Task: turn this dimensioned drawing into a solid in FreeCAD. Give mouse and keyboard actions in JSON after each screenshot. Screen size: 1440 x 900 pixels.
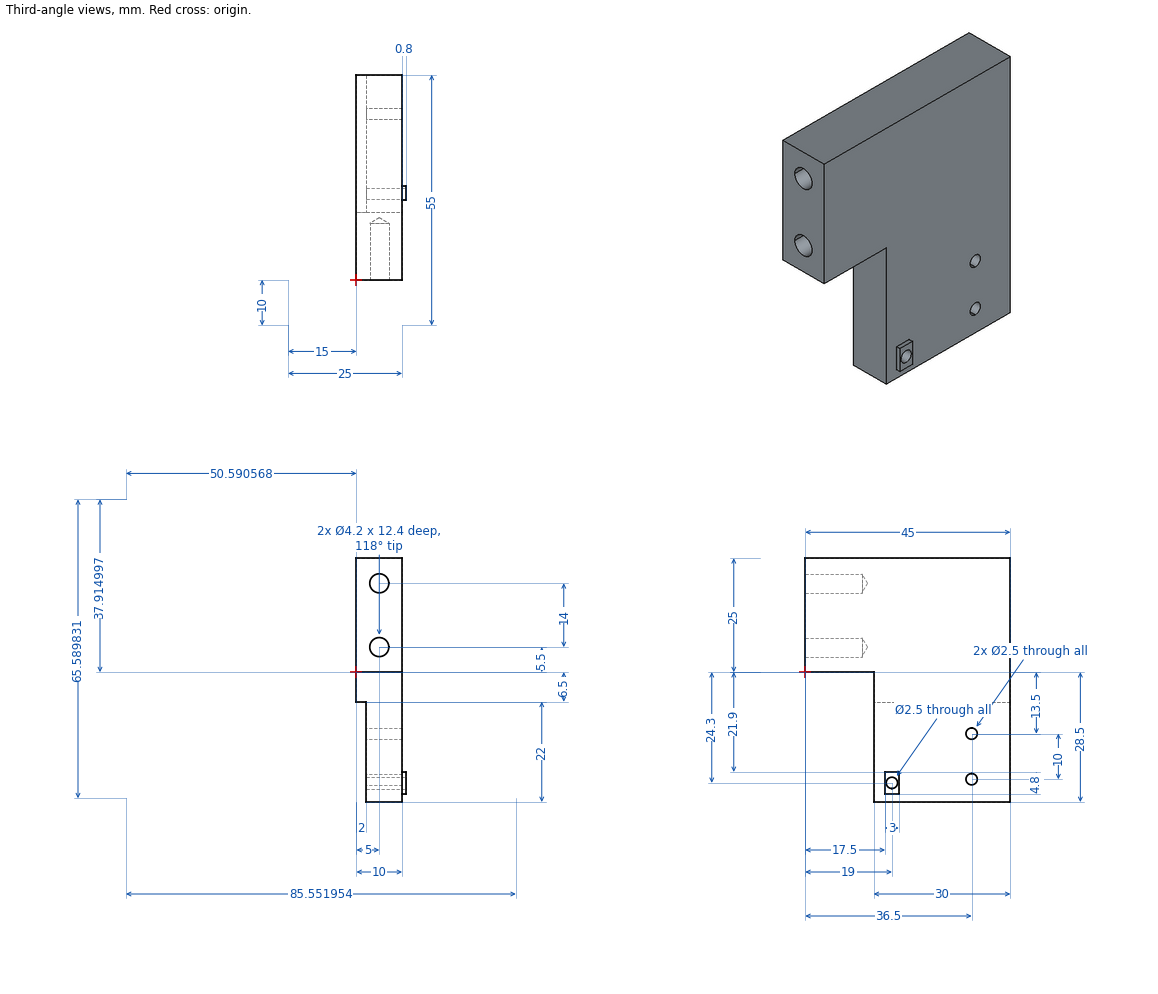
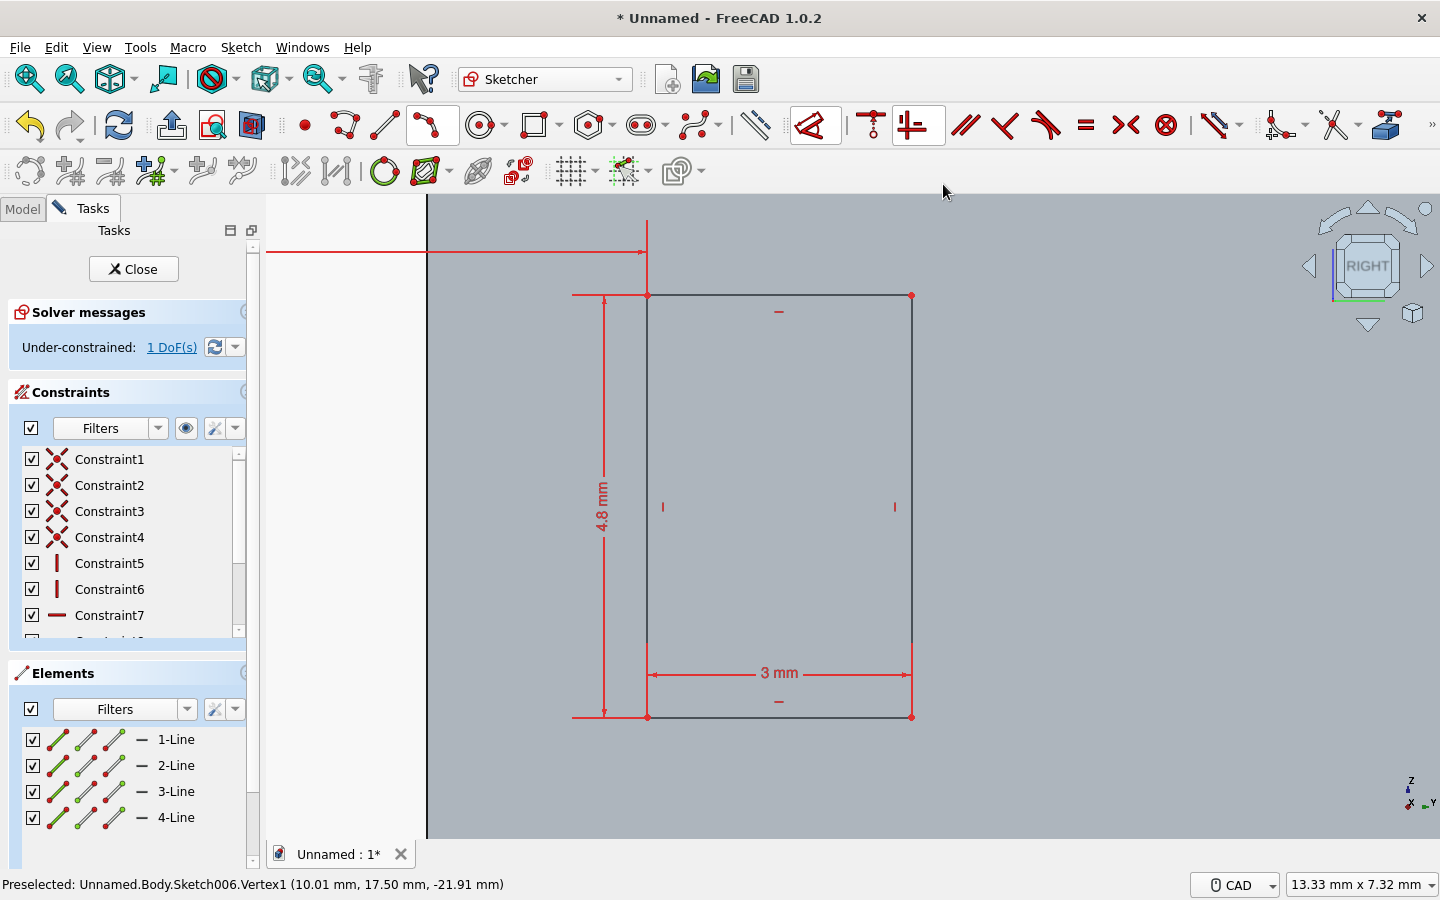
{"action": "left_click", "coordinate": [647, 295]}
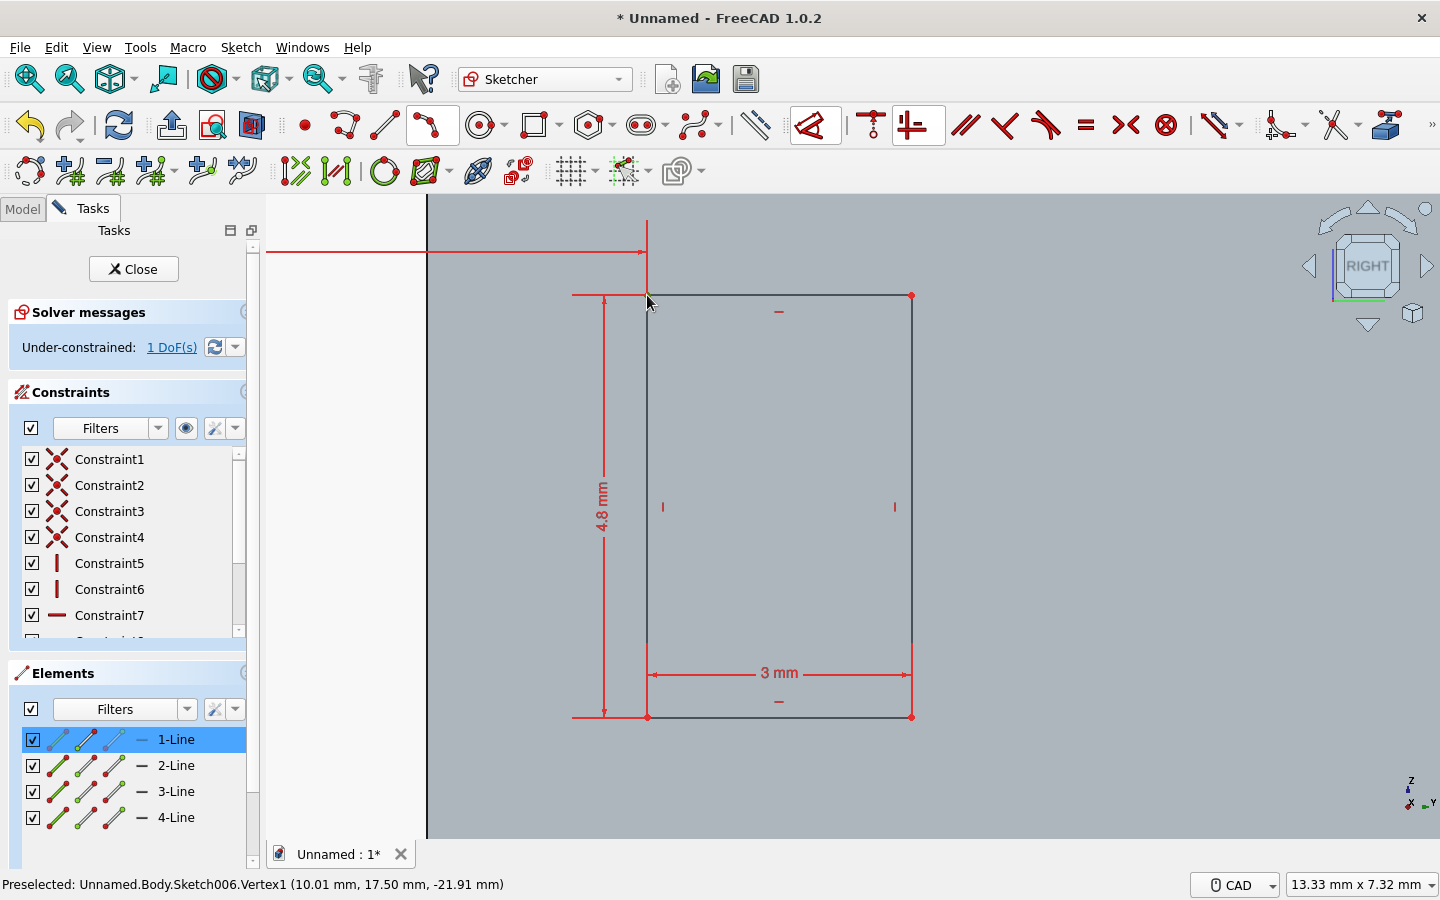
{"action": "key", "text": "i"}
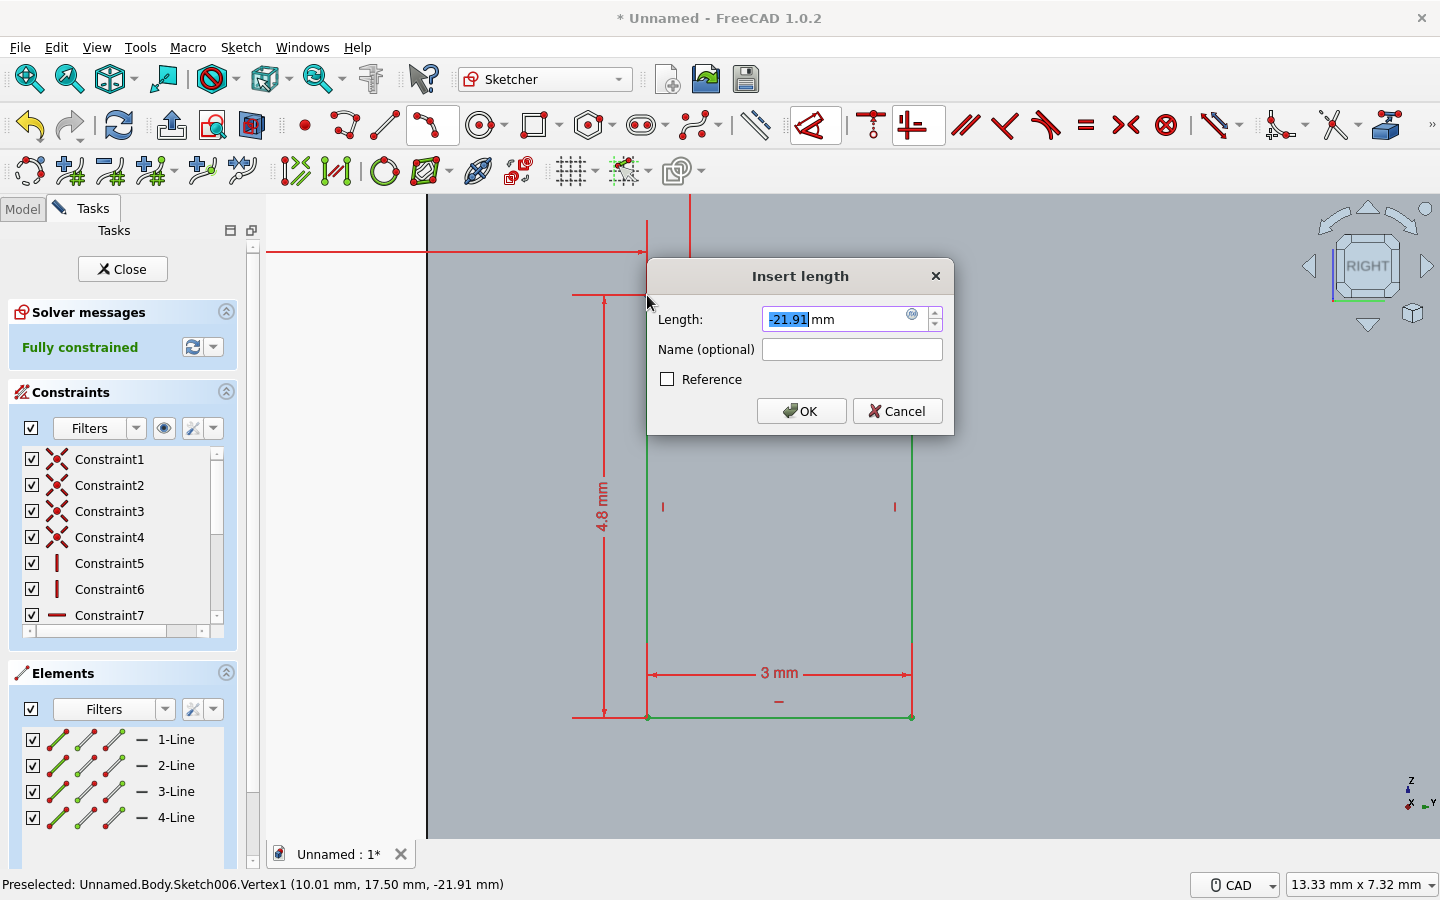
{"action": "type", "text": "-21.9"}
{"action": "key", "text": "Return"}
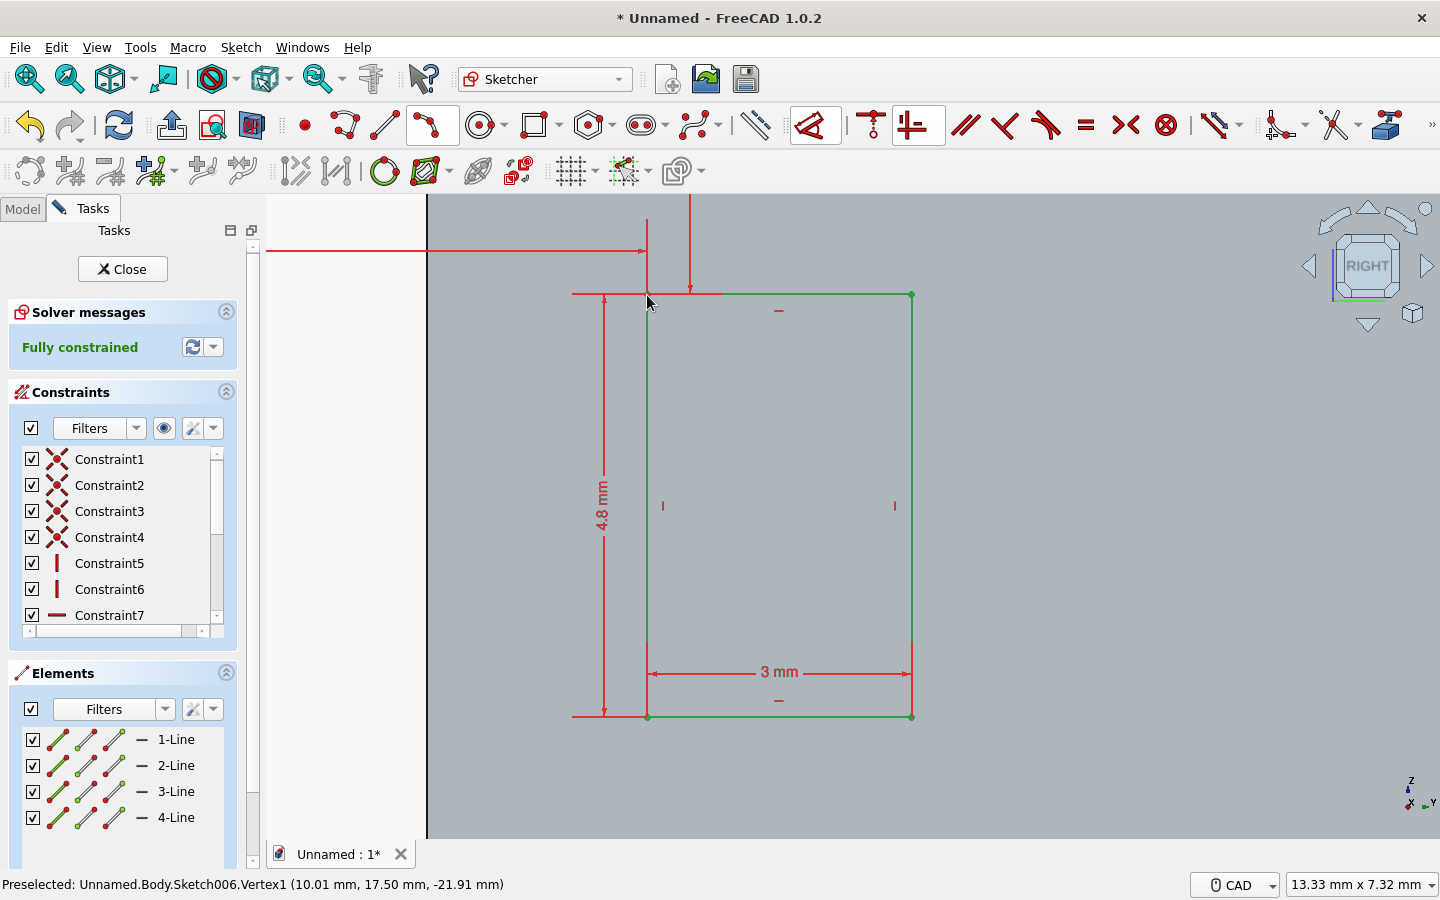
{"action": "left_click", "coordinate": [123, 269]}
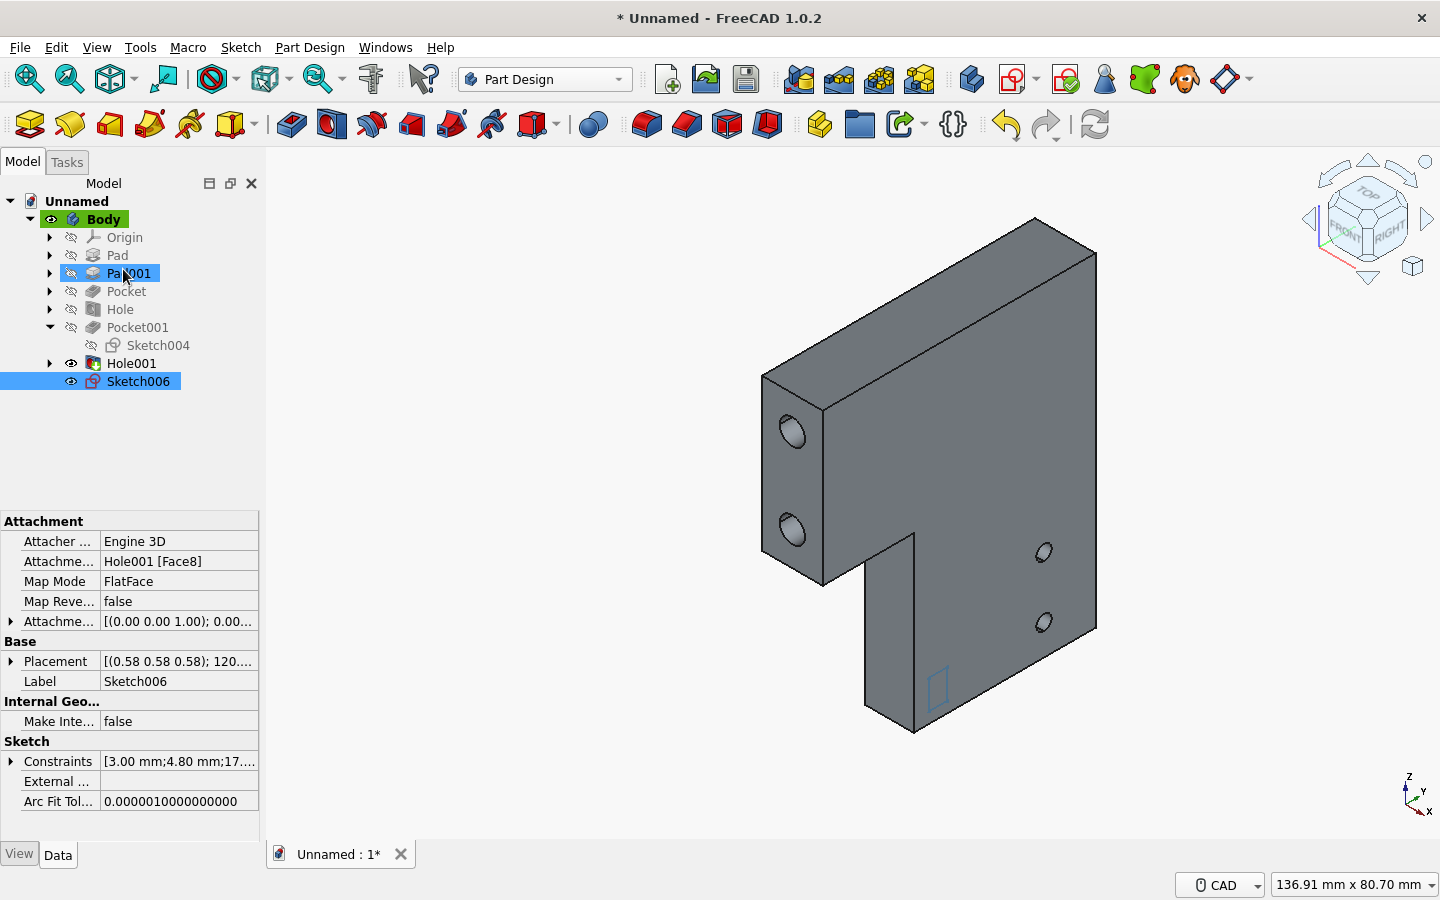
{"action": "left_click", "coordinate": [30, 124]}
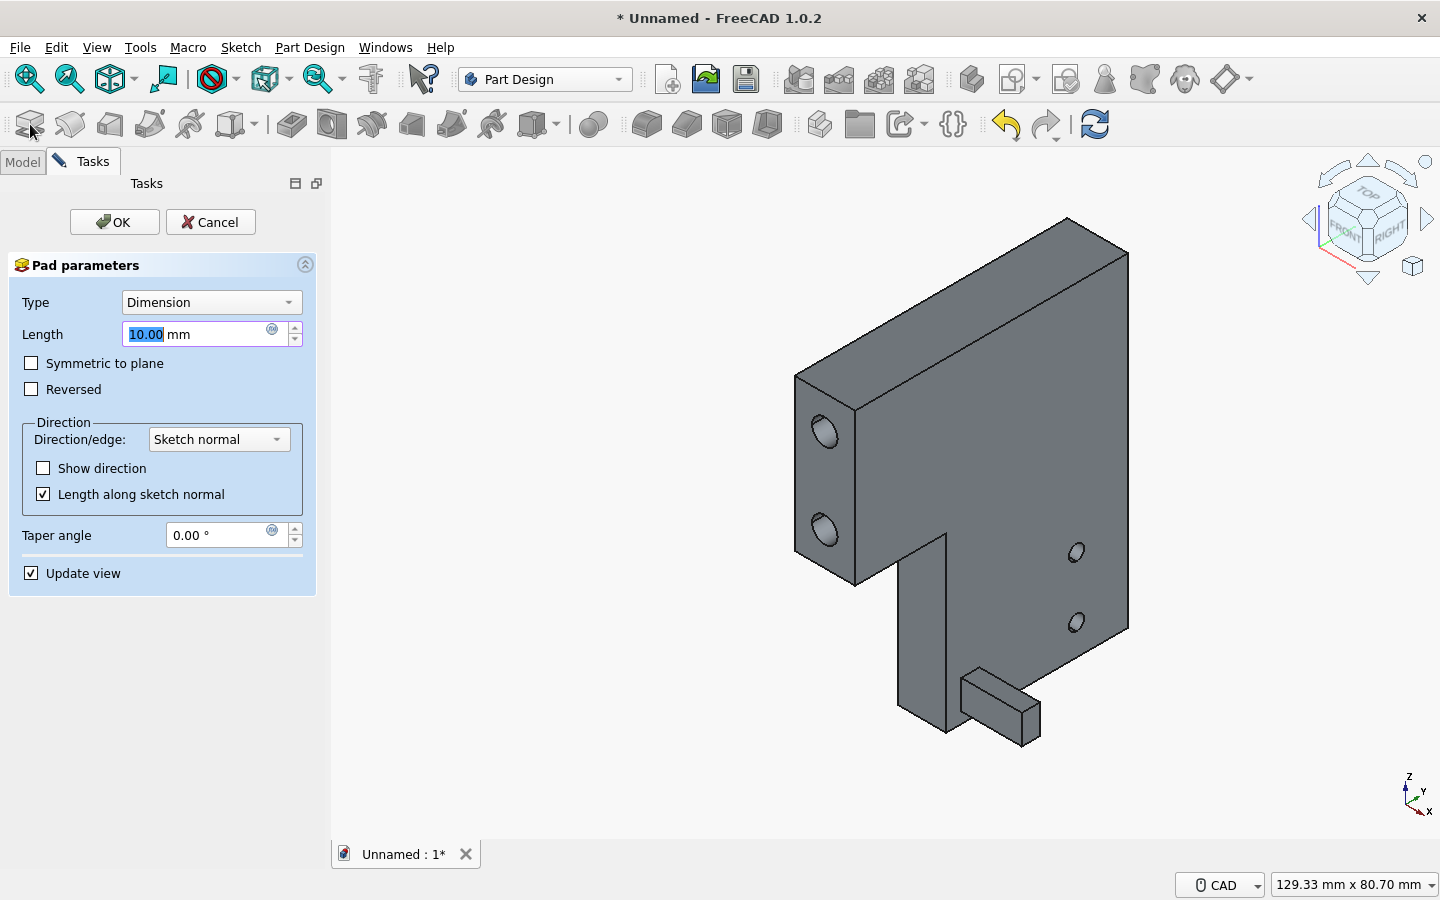
{"action": "type", "text": "0.8"}
{"action": "key", "text": "Tab"}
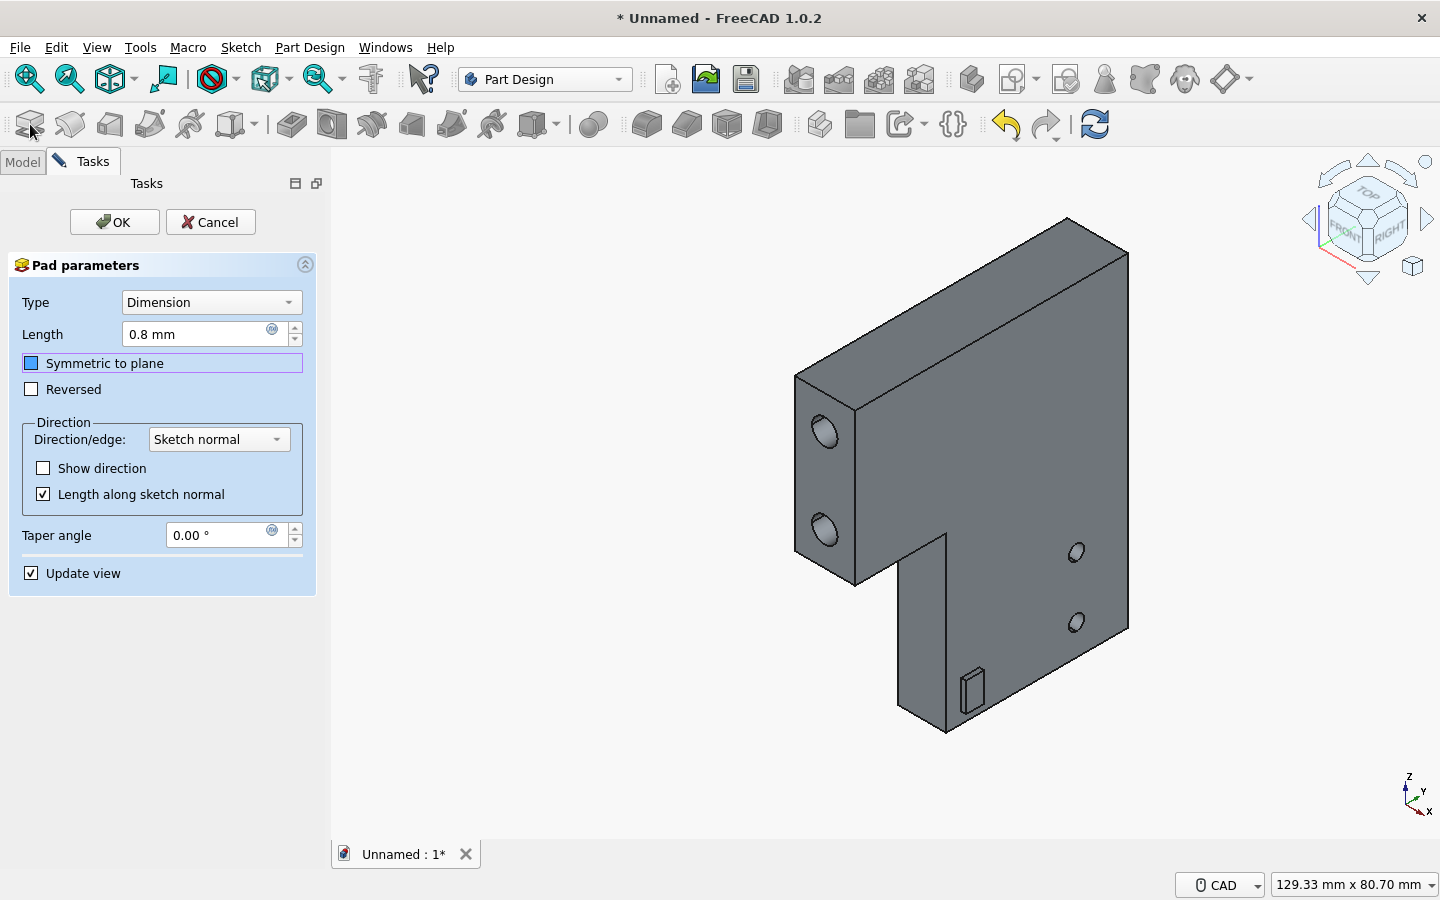
{"action": "left_click", "coordinate": [115, 222]}